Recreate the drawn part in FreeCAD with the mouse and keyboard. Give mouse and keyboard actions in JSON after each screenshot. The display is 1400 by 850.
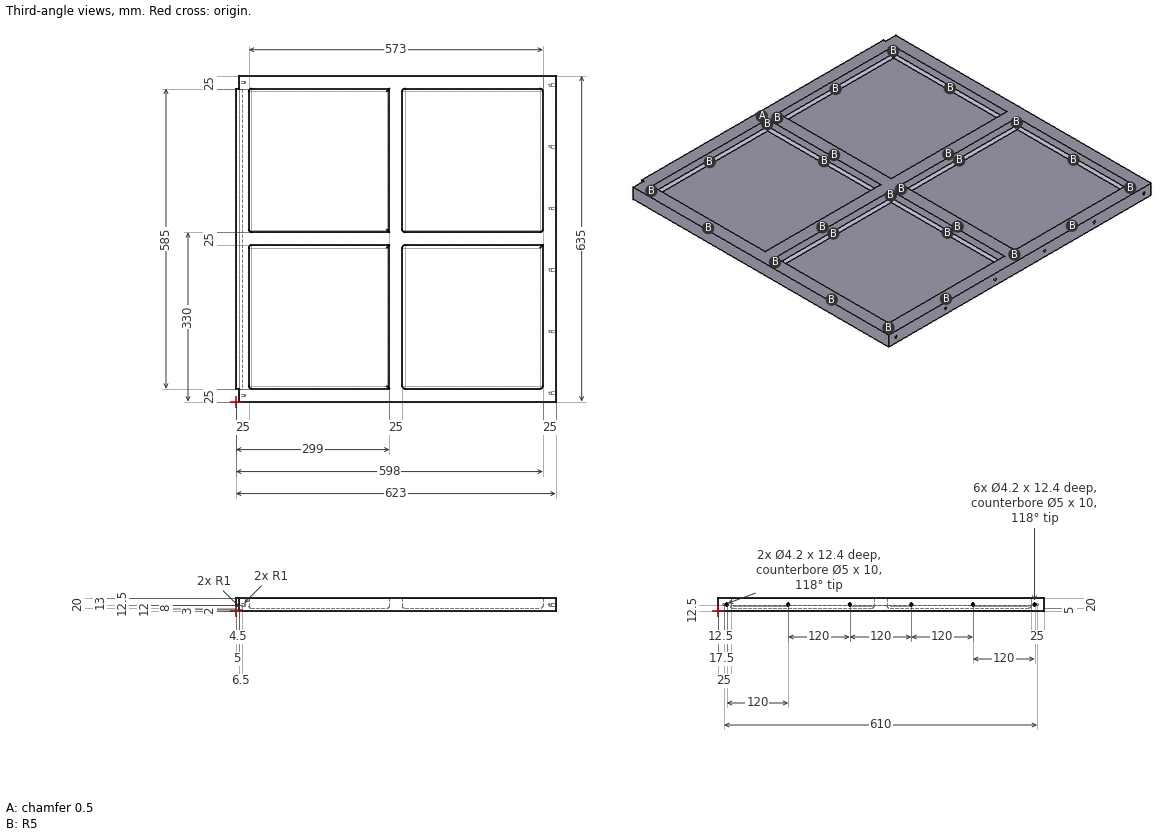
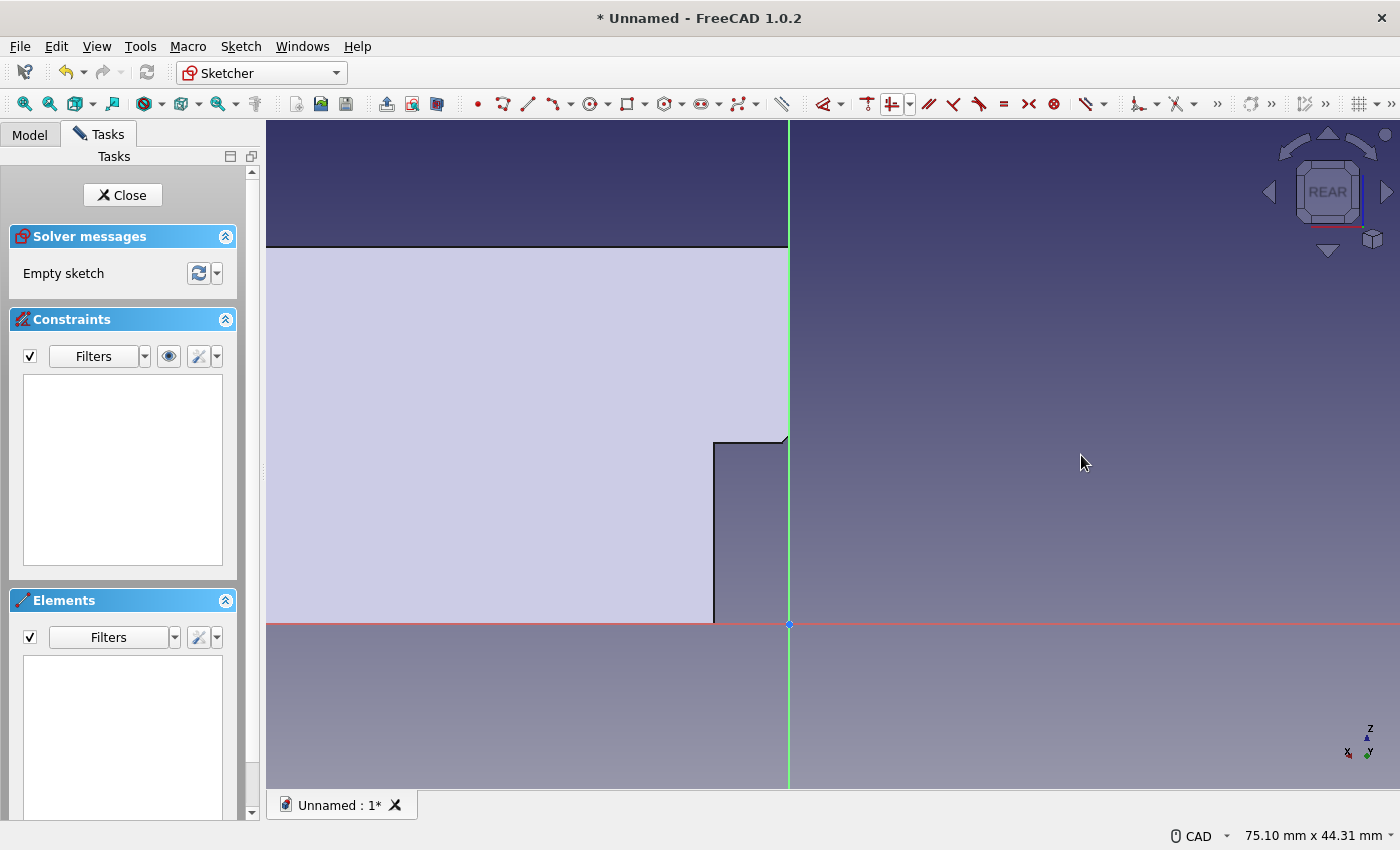
{"action": "left_click", "coordinate": [503, 104]}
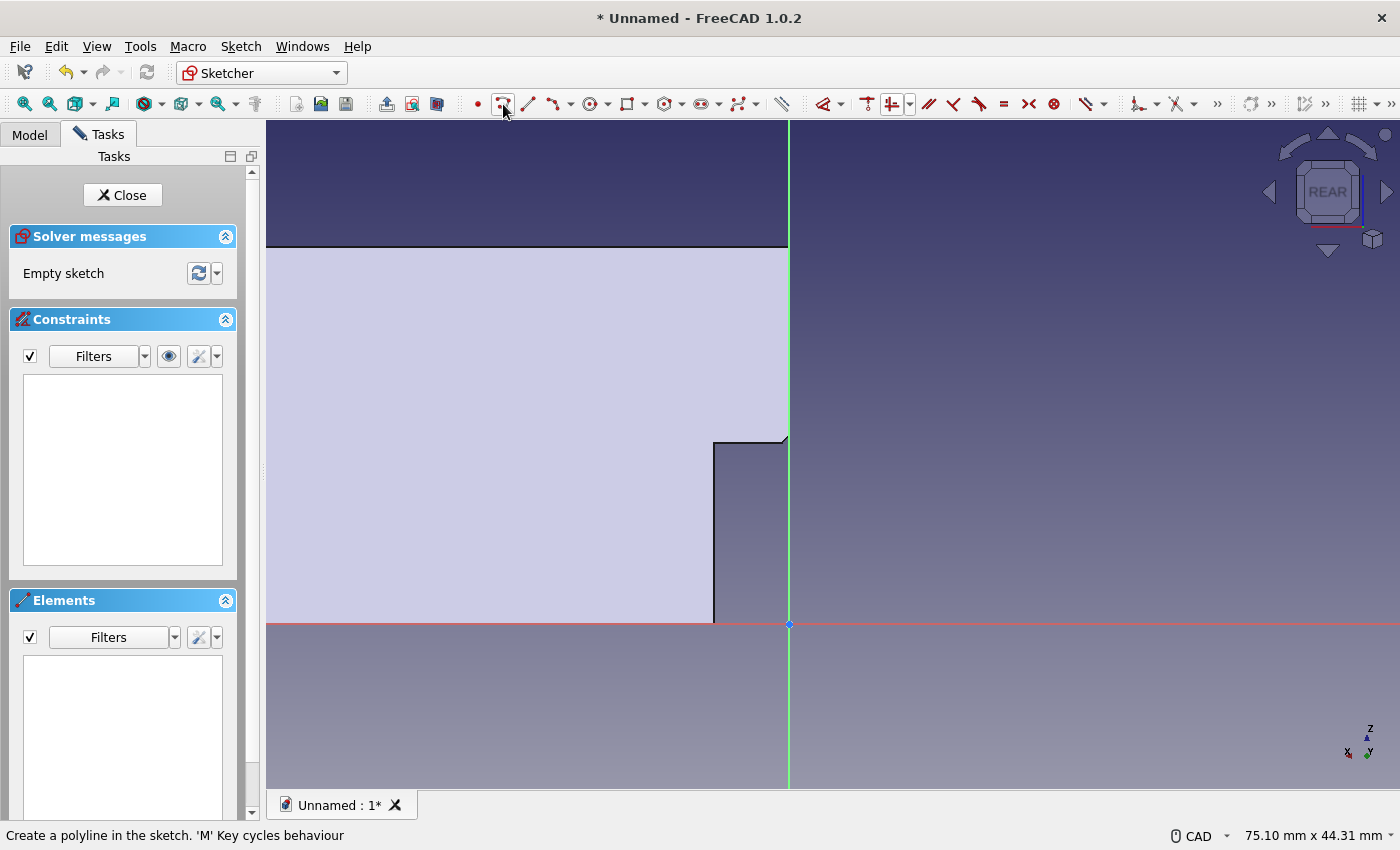
{"action": "scroll", "coordinate": [782, 443], "scroll_direction": "up", "scroll_amount": 4}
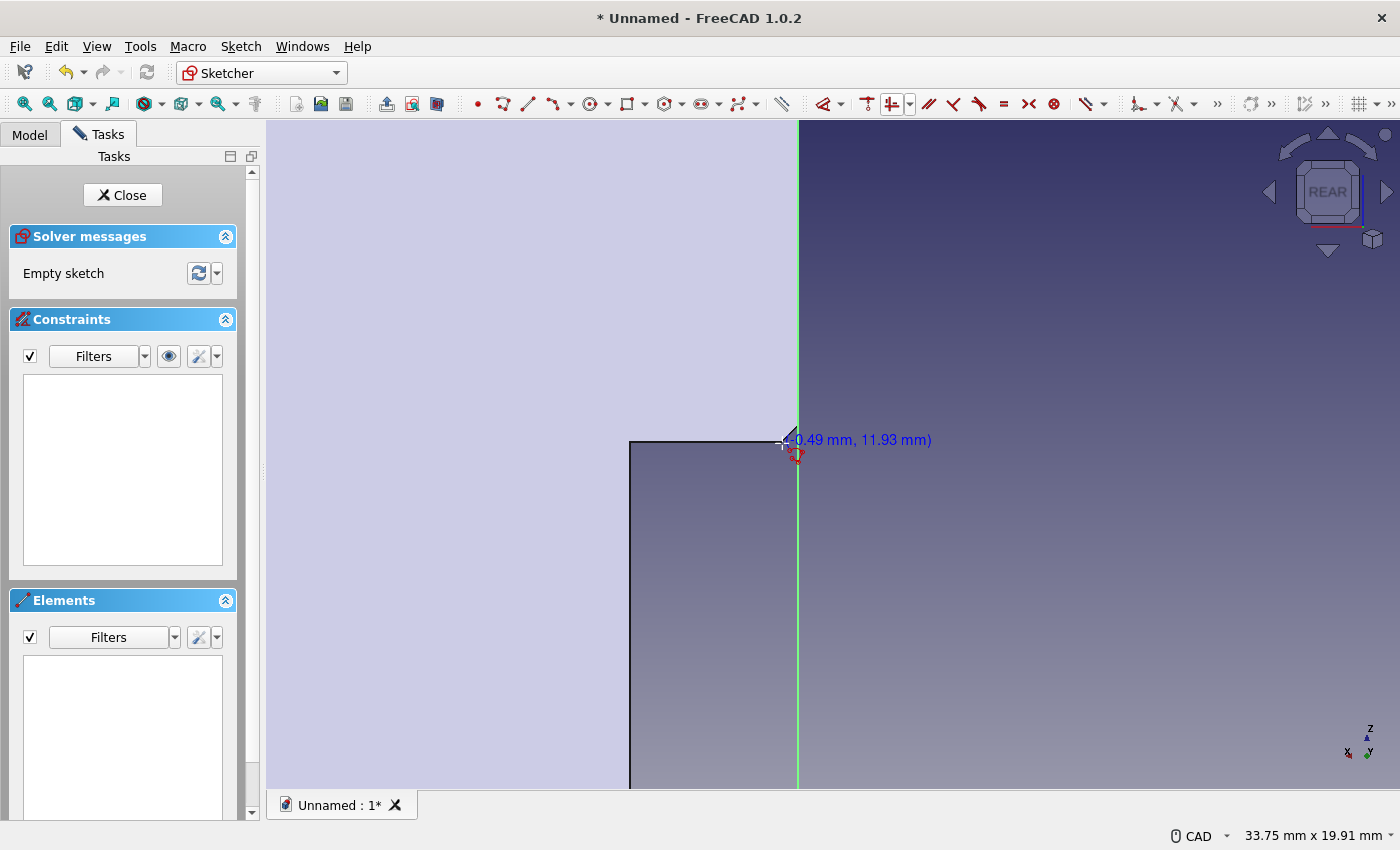
{"action": "left_click", "coordinate": [781, 442]}
{"action": "left_click", "coordinate": [798, 425]}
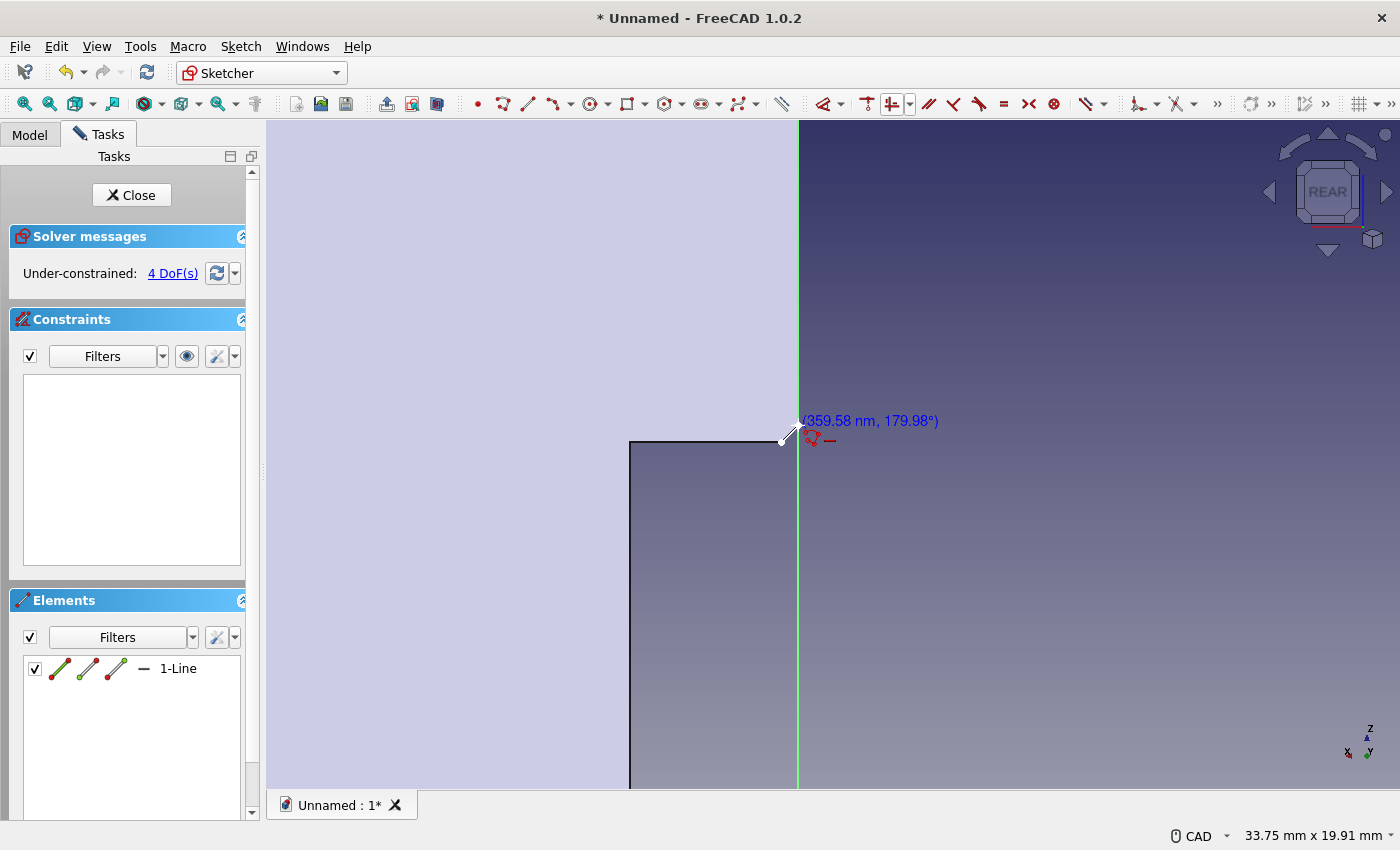
{"action": "scroll", "coordinate": [826, 490], "scroll_direction": "down", "scroll_amount": 3}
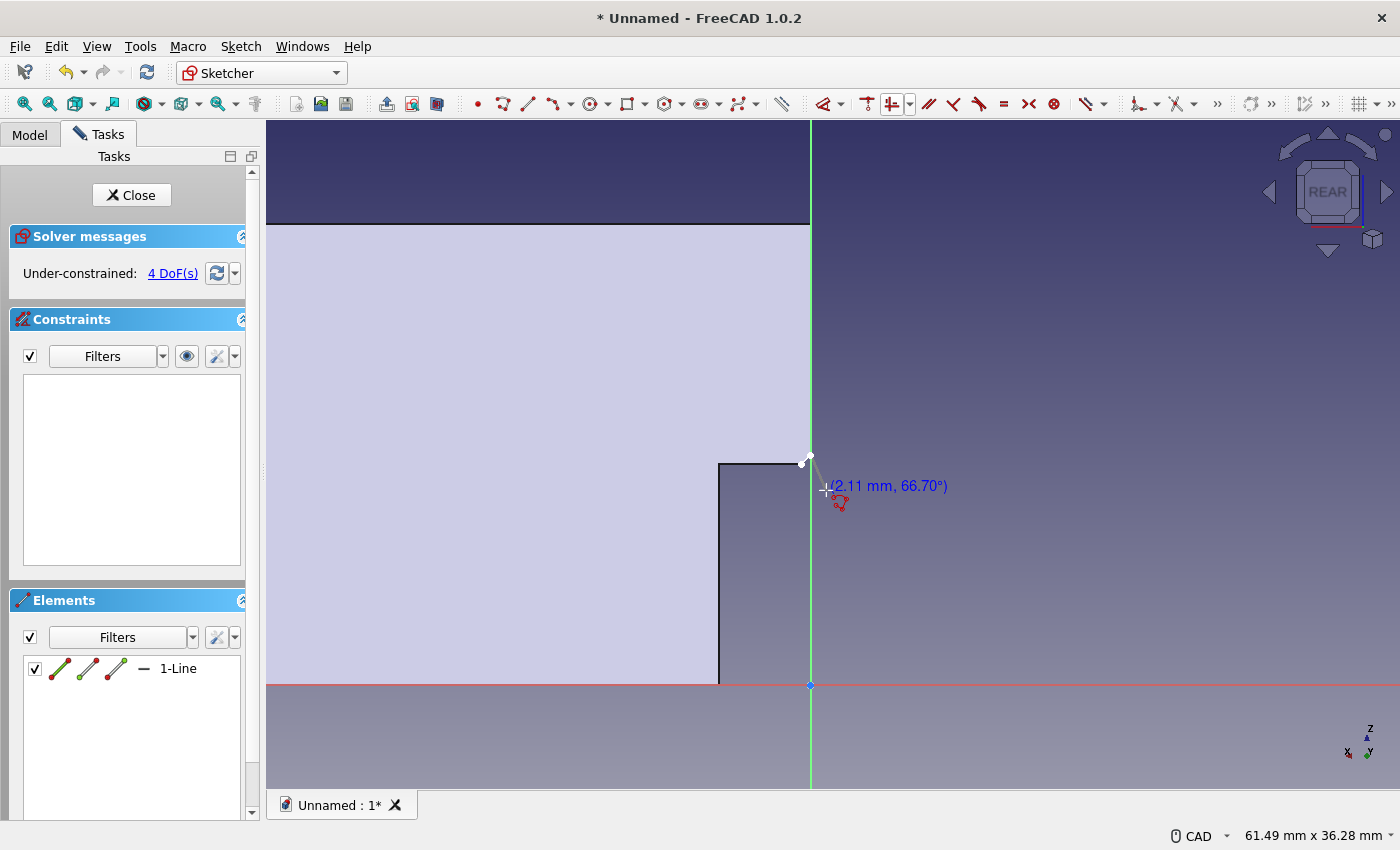
{"action": "left_click", "coordinate": [802, 224]}
{"action": "left_click", "coordinate": [719, 224]}
{"action": "left_click", "coordinate": [719, 464]}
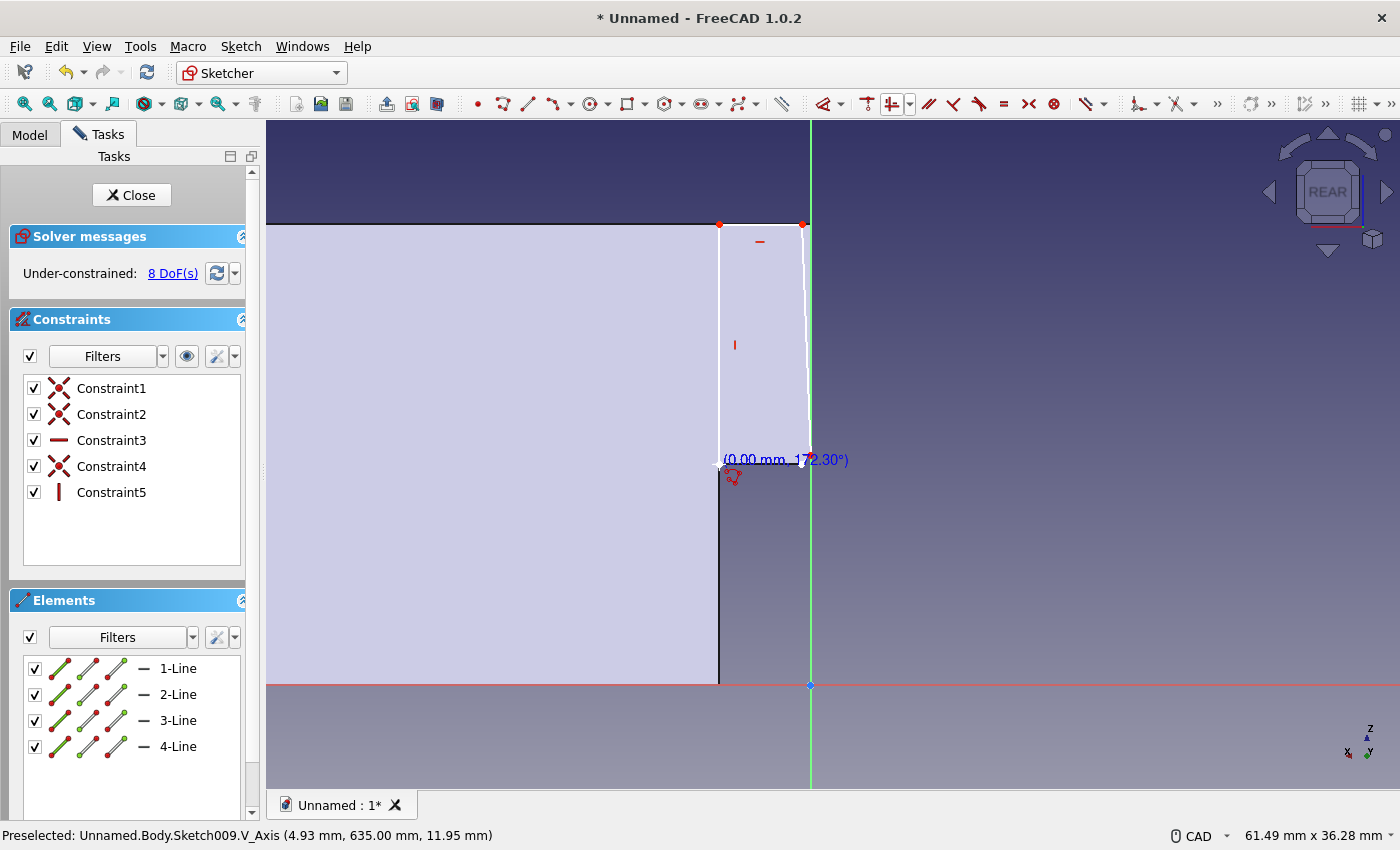
{"action": "scroll", "coordinate": [802, 464], "scroll_direction": "up", "scroll_amount": 5}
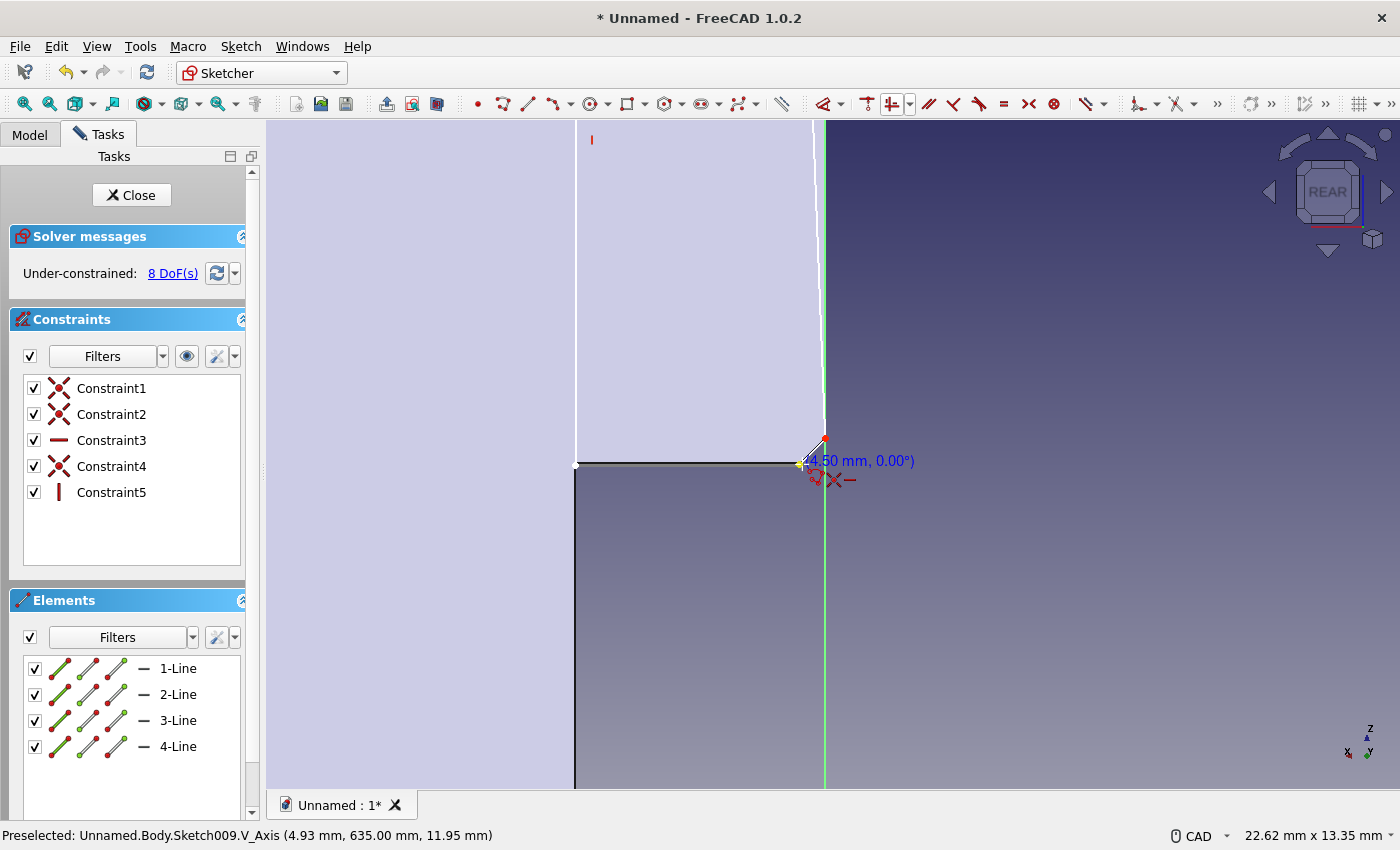
{"action": "left_click", "coordinate": [800, 464]}
{"action": "key", "text": "Escape"}
{"action": "key", "text": "Escape"}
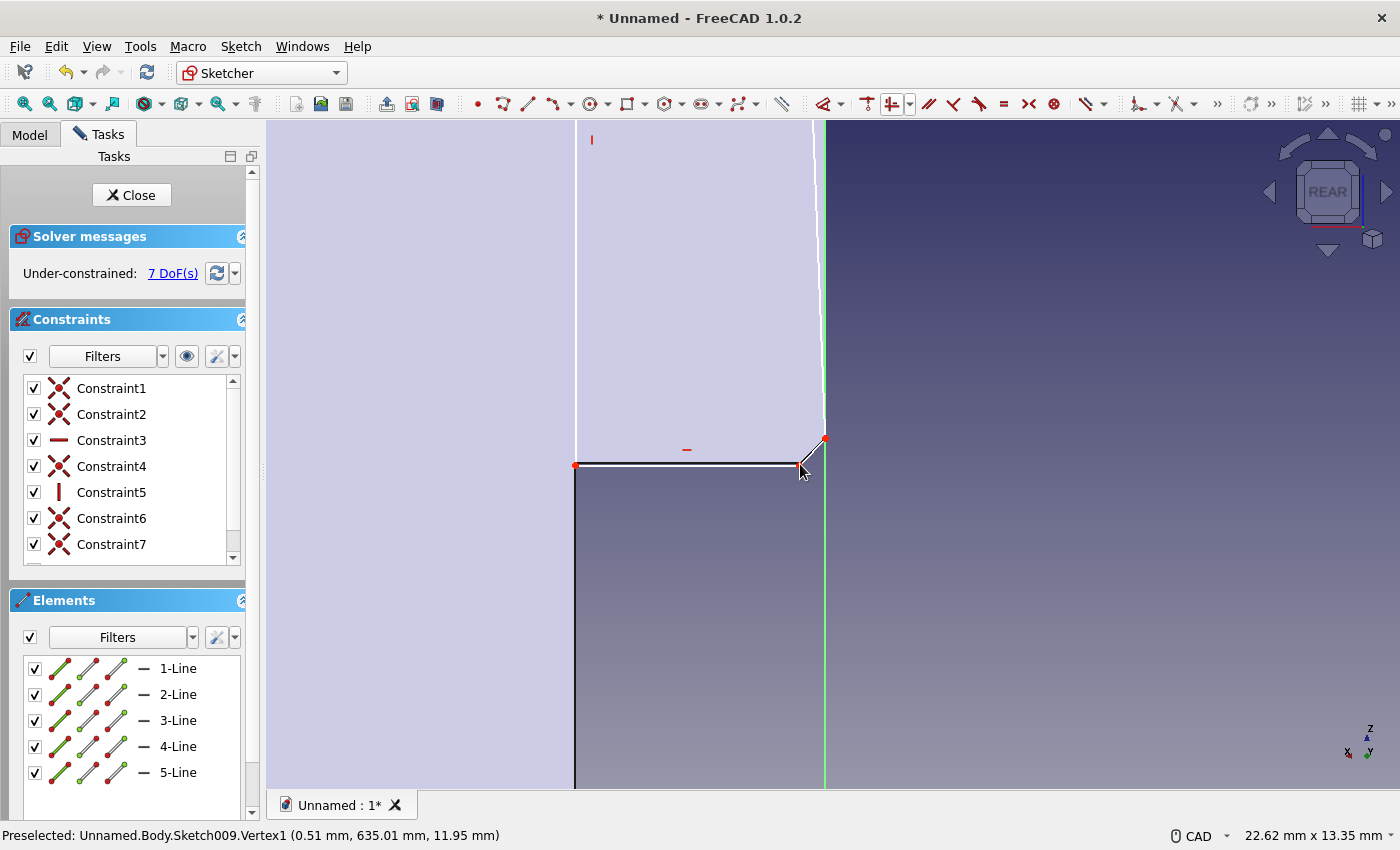
{"action": "scroll", "coordinate": [816, 189], "scroll_direction": "up", "scroll_amount": 2}